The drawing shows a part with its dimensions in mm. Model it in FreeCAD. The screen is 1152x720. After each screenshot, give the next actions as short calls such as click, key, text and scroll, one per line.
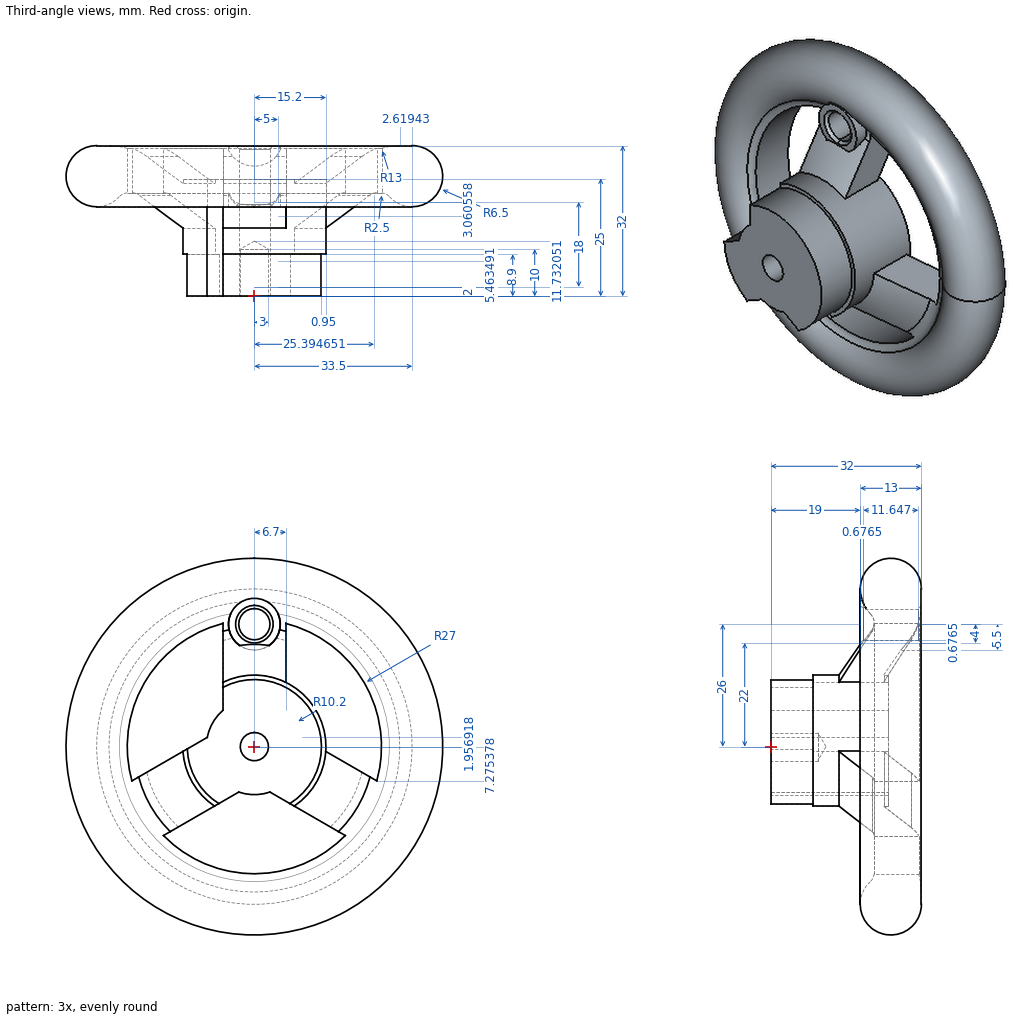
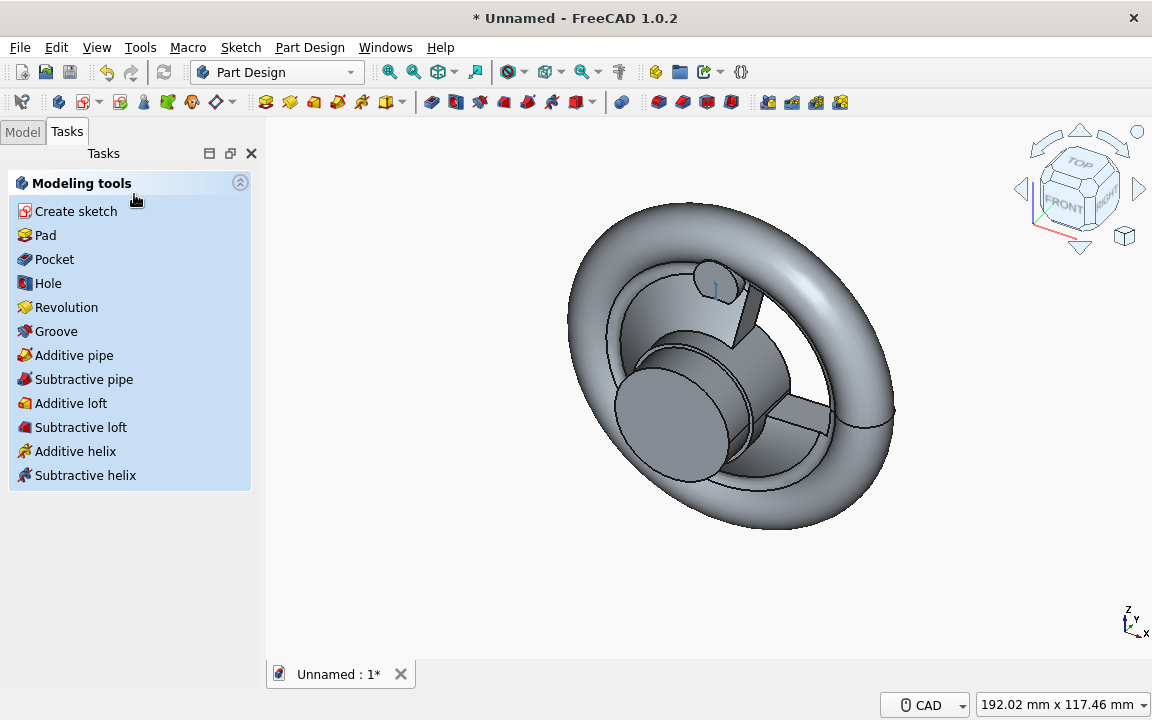
click(480, 102)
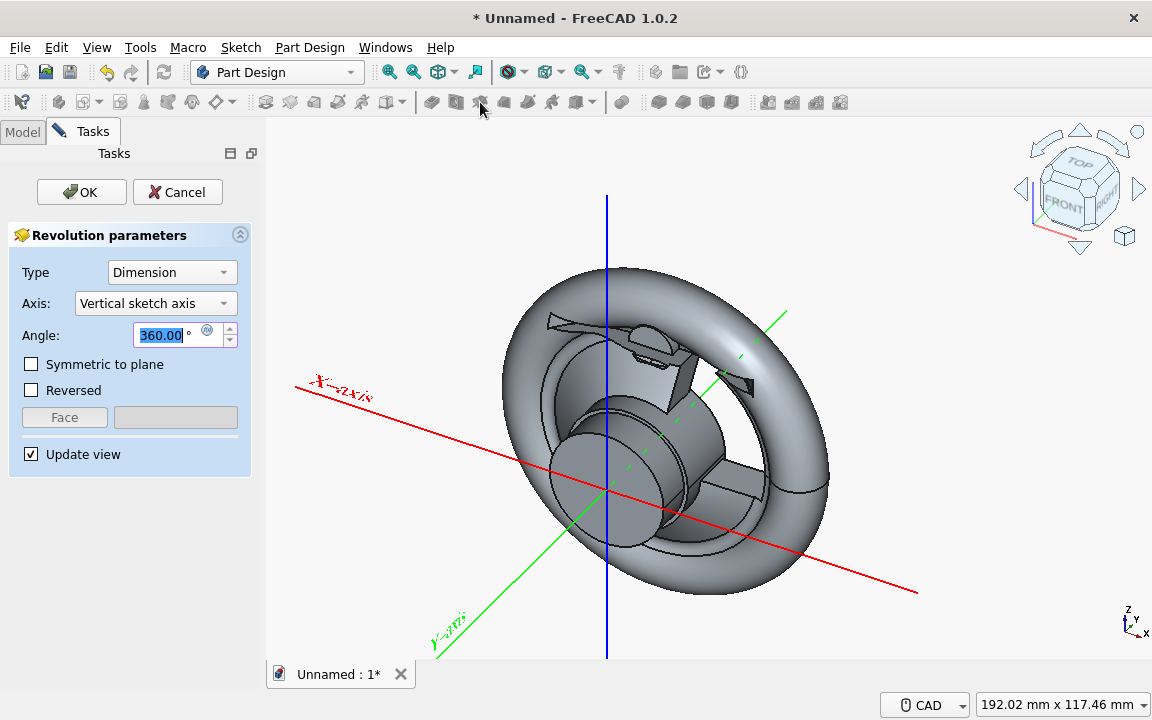
click(156, 304)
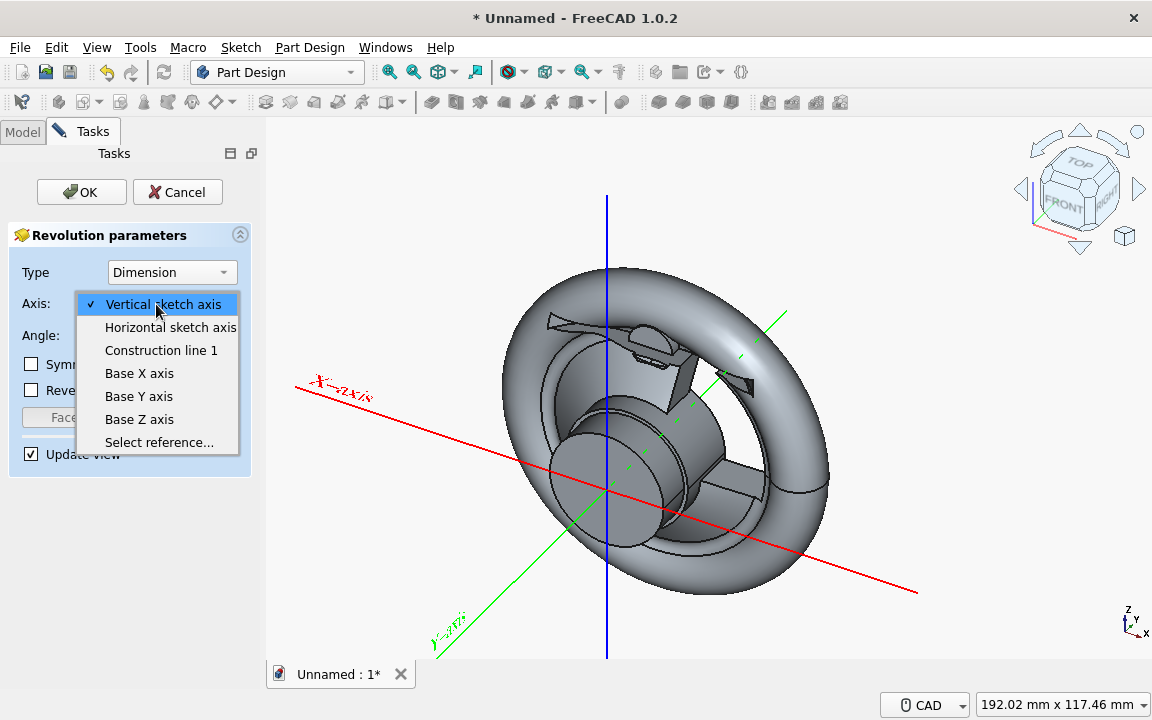
click(156, 350)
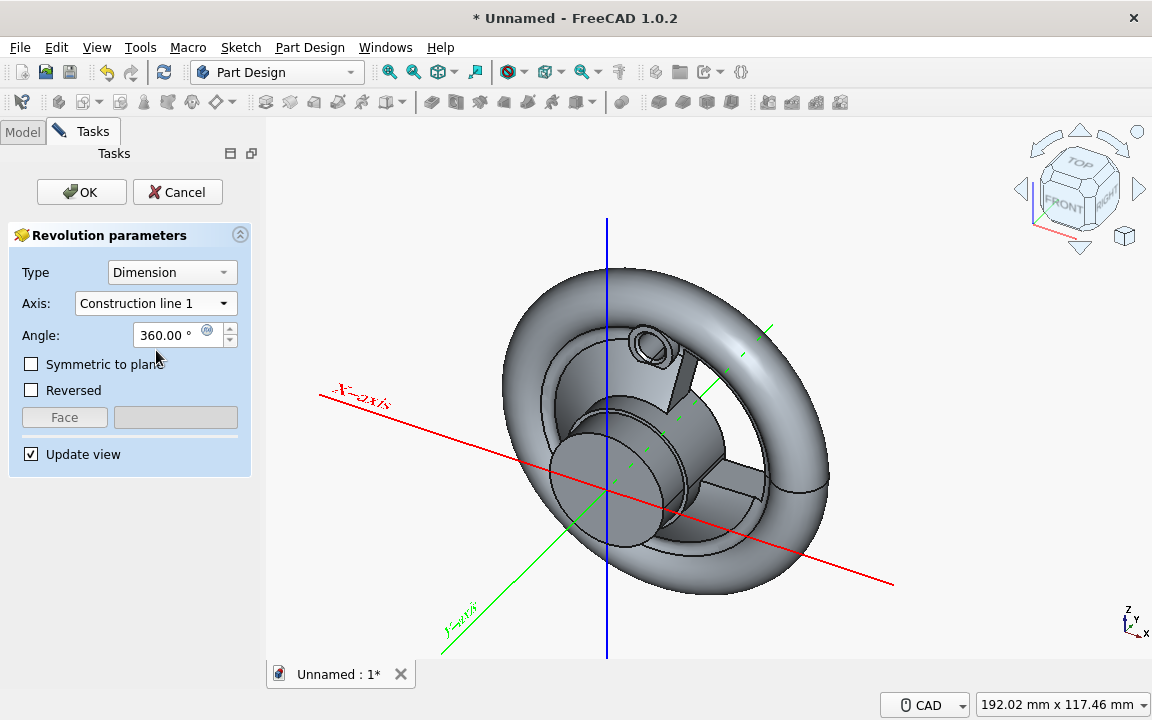
click(82, 192)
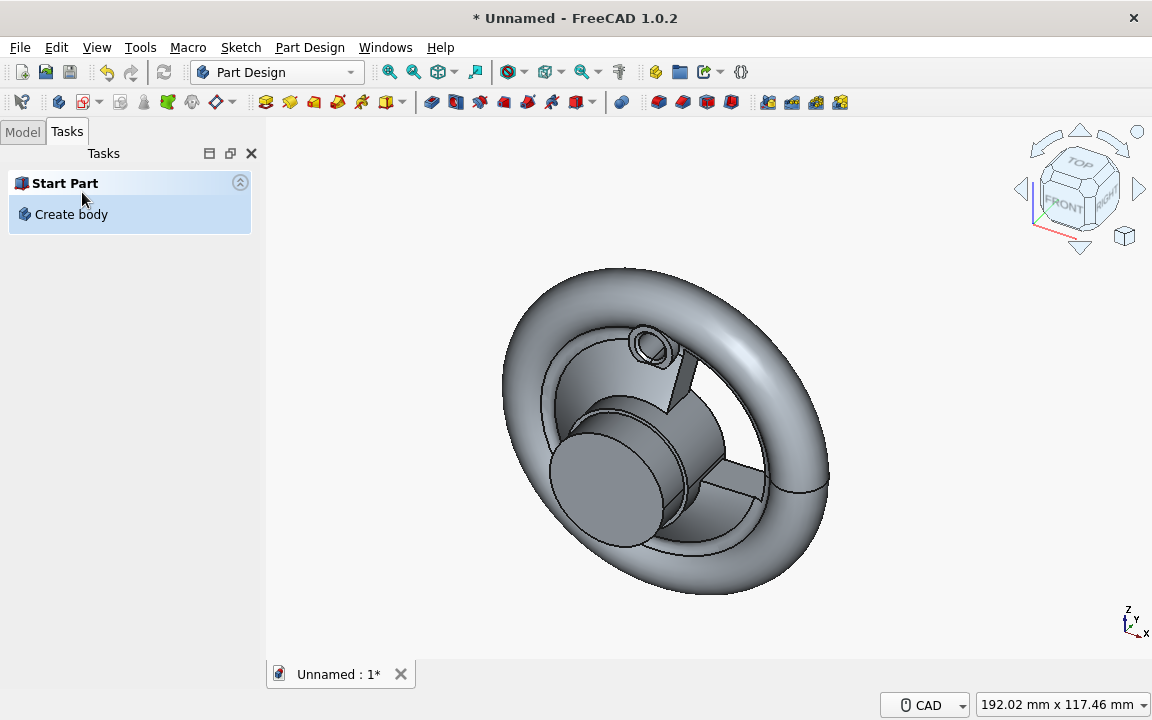
click(390, 72)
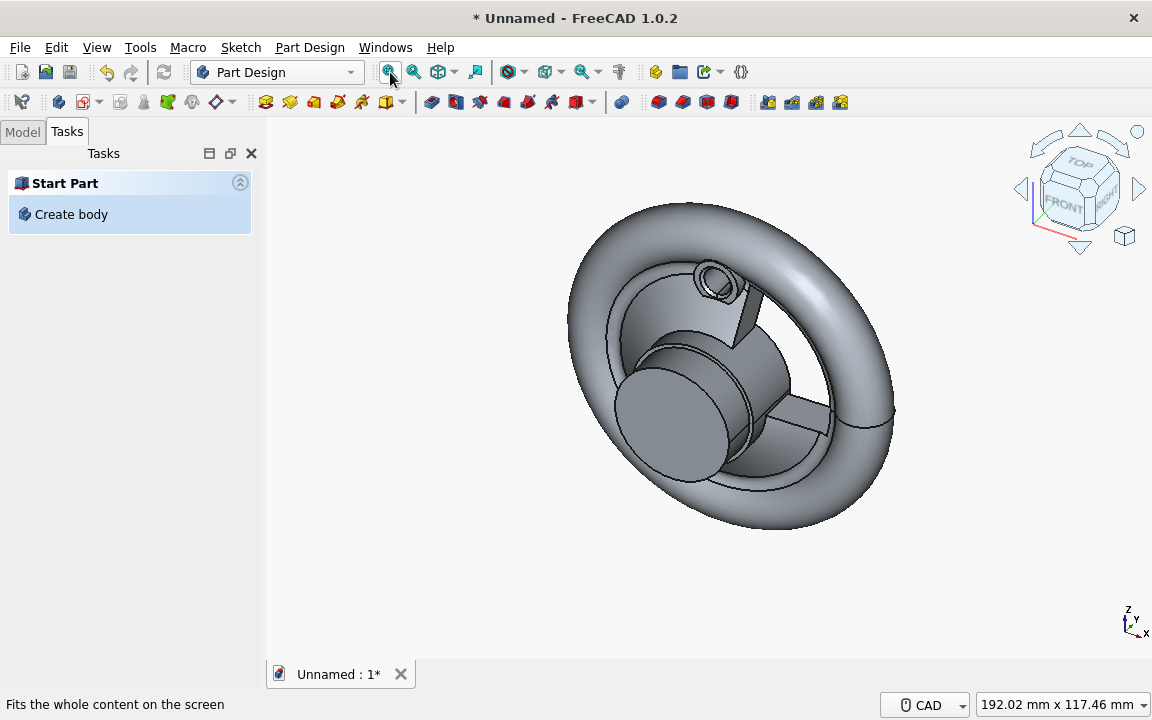
click(84, 102)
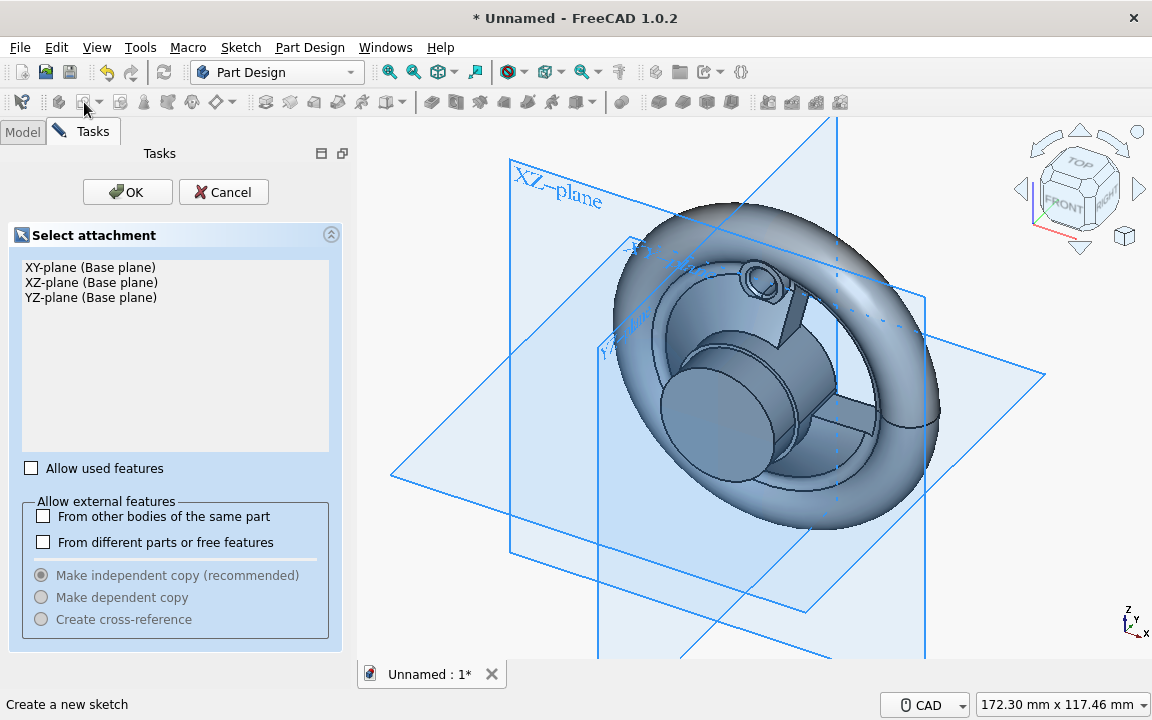
click(82, 268)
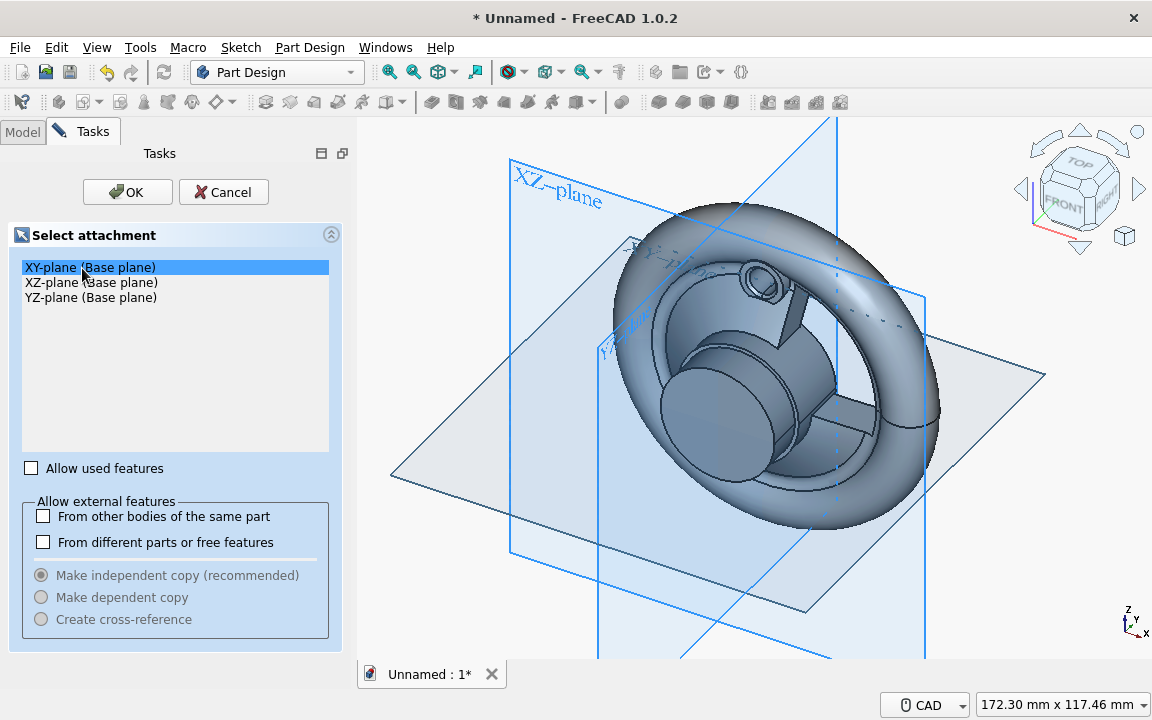
click(128, 192)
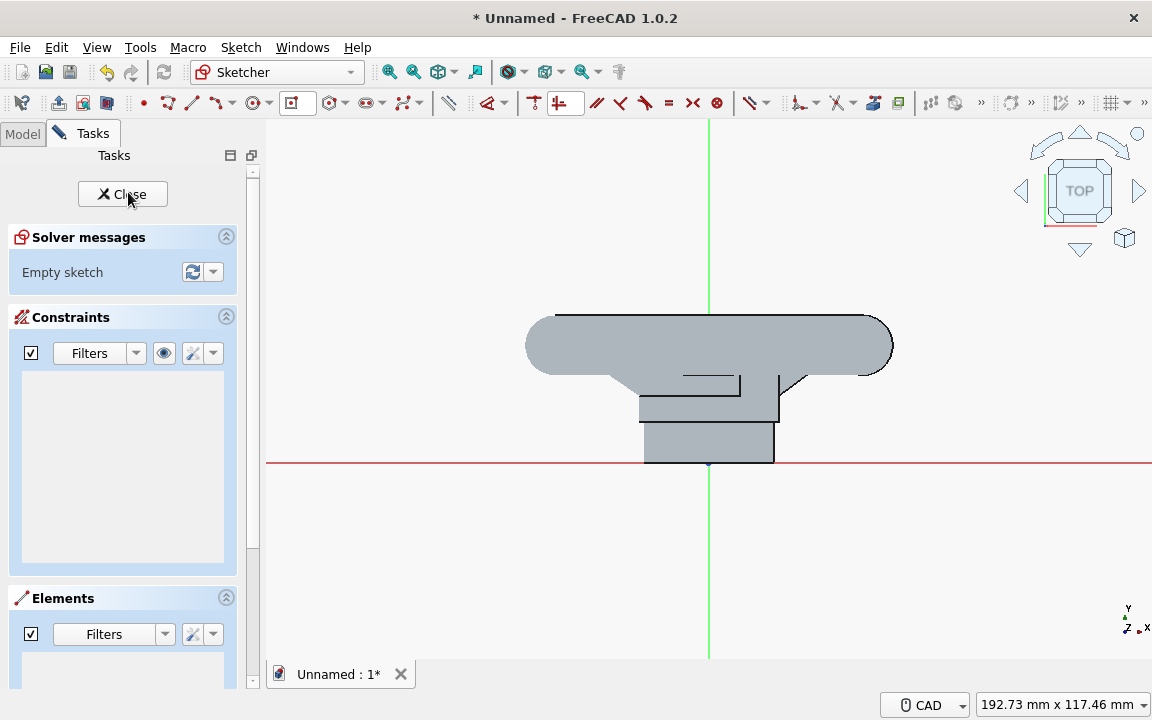
click(108, 104)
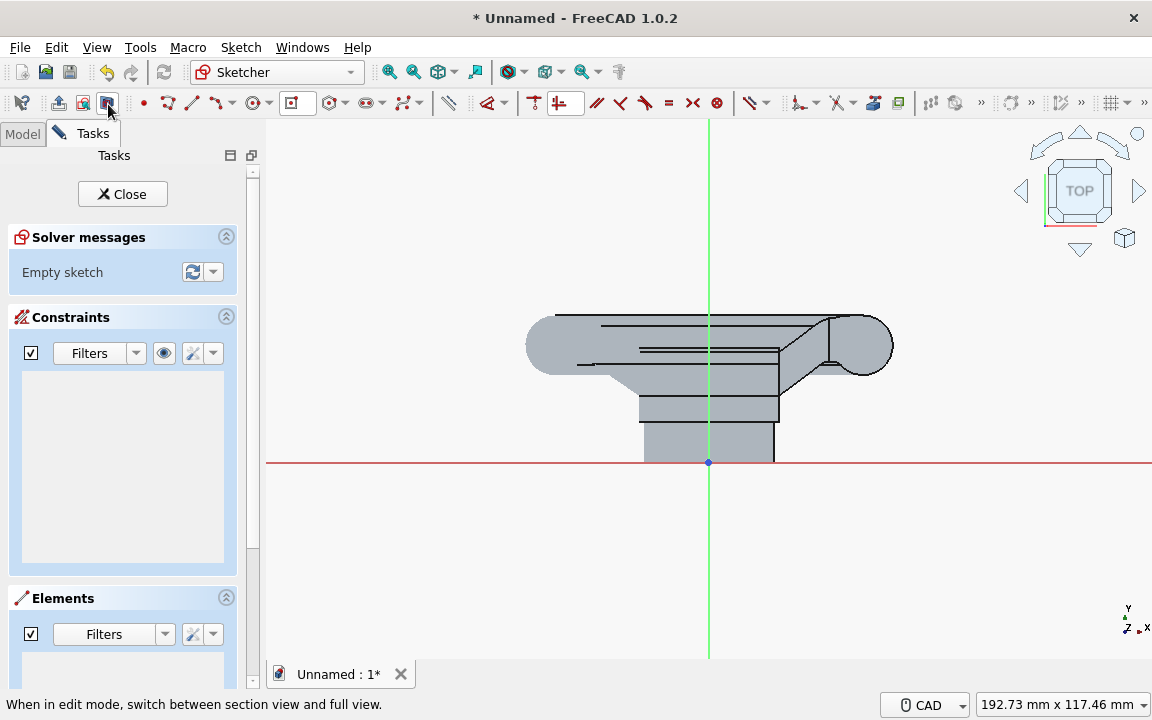
scroll(731, 445, up, 9)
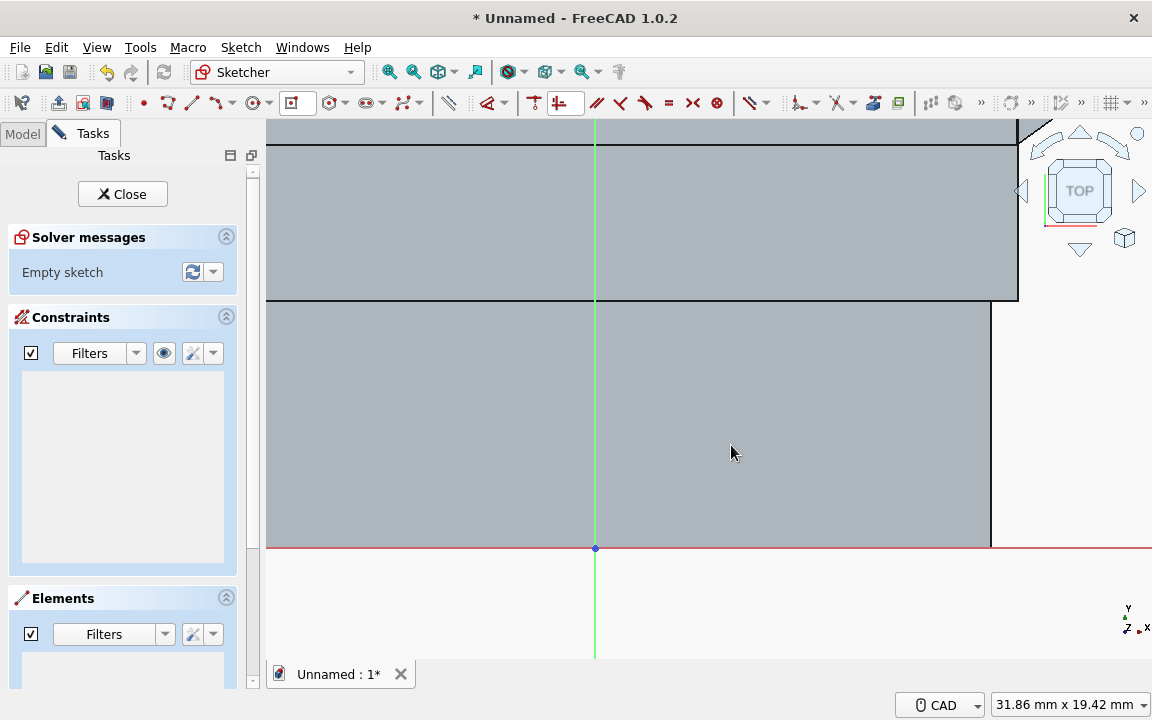
click(168, 104)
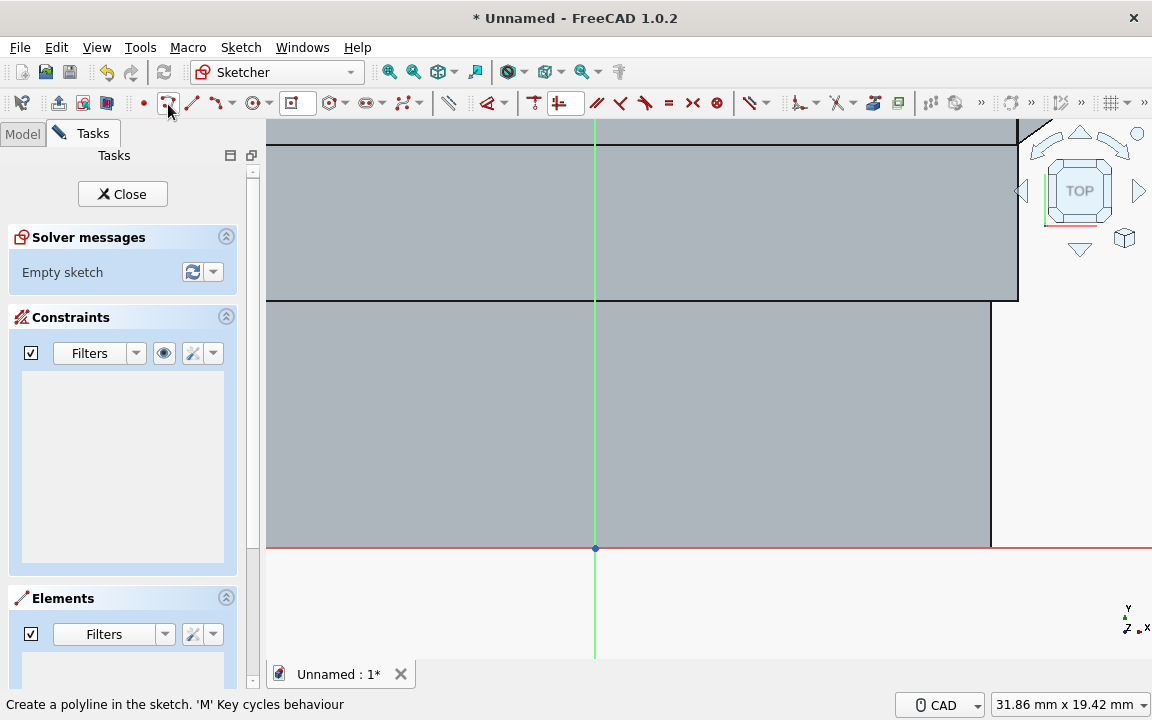
click(595, 548)
click(679, 539)
click(679, 270)
click(604, 222)
click(595, 548)
key(Escape)
key(Escape)